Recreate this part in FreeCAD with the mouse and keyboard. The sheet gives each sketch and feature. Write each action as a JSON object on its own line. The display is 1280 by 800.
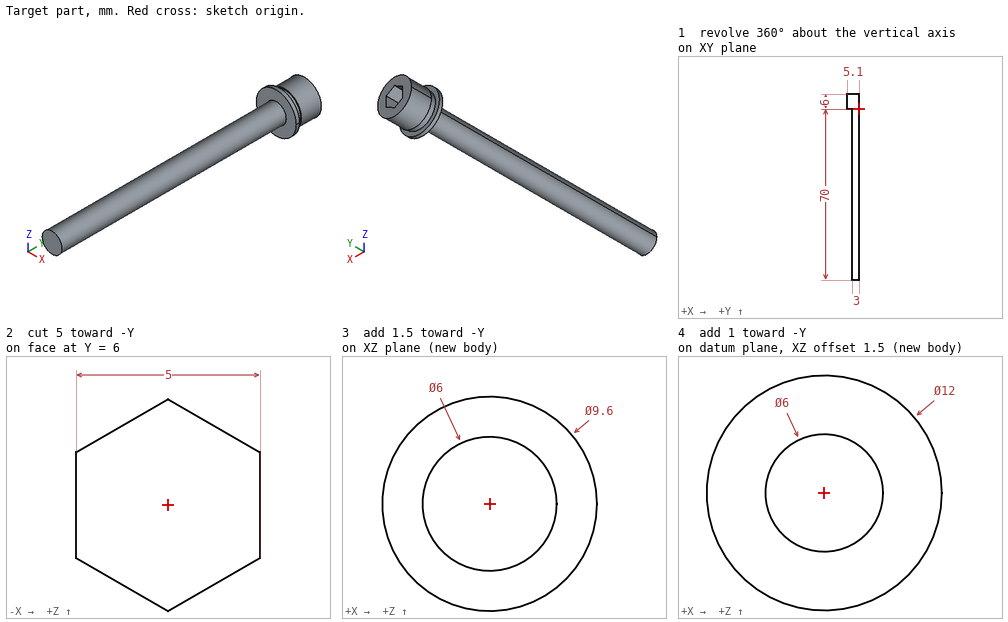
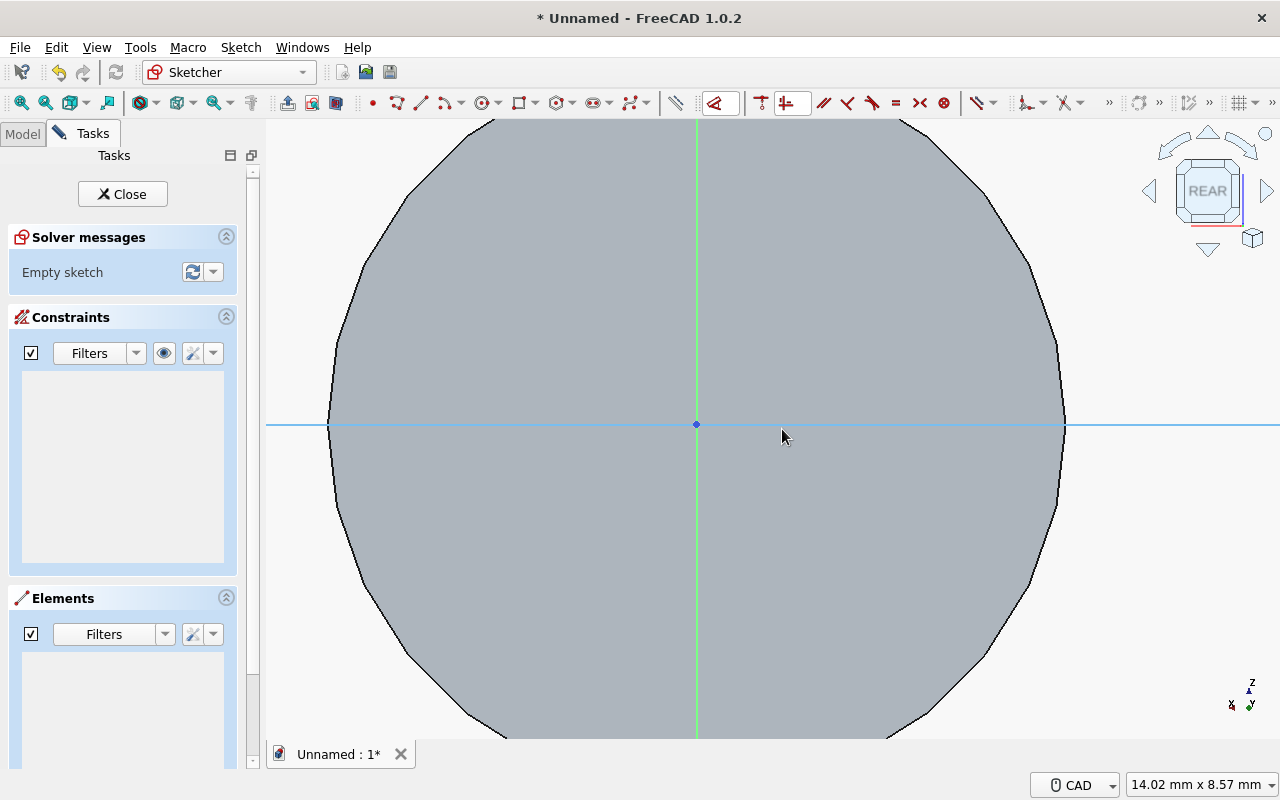
{"action": "key", "text": "g p 6"}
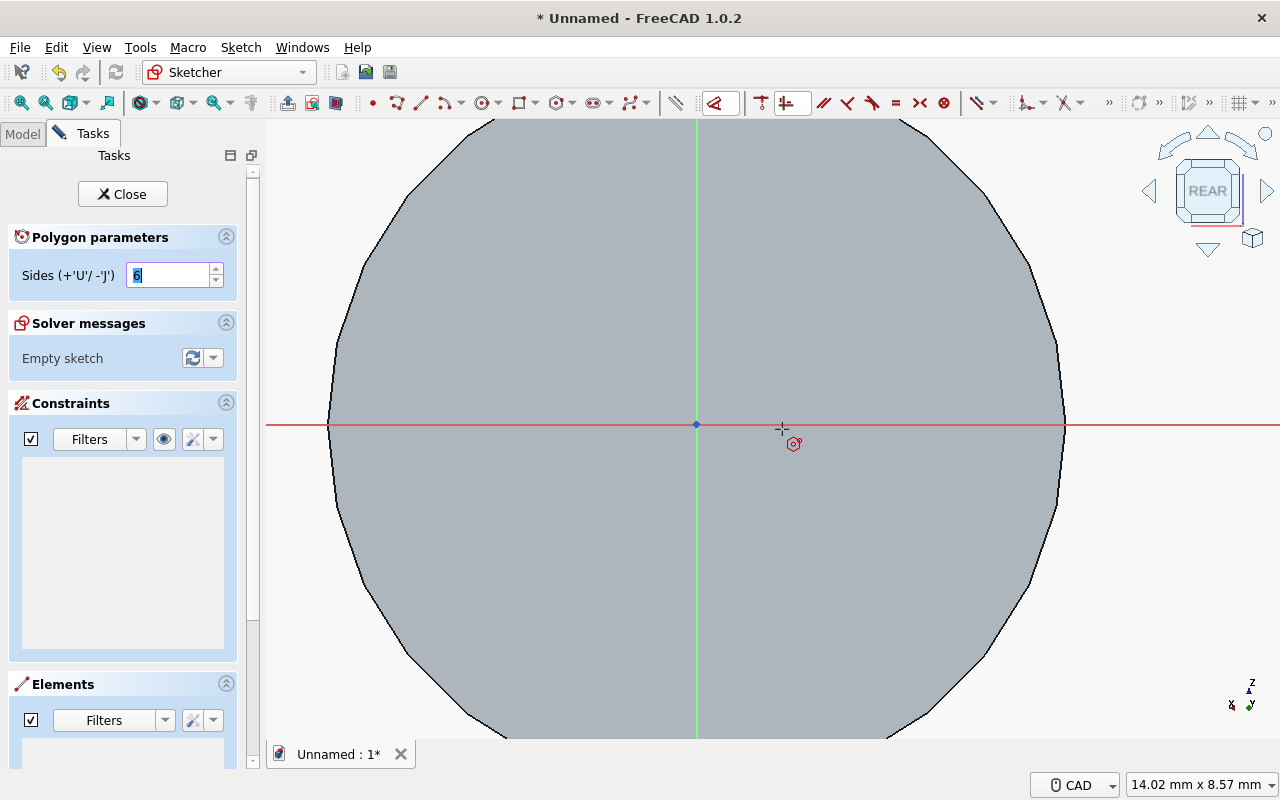
{"action": "left_click", "coordinate": [697, 425]}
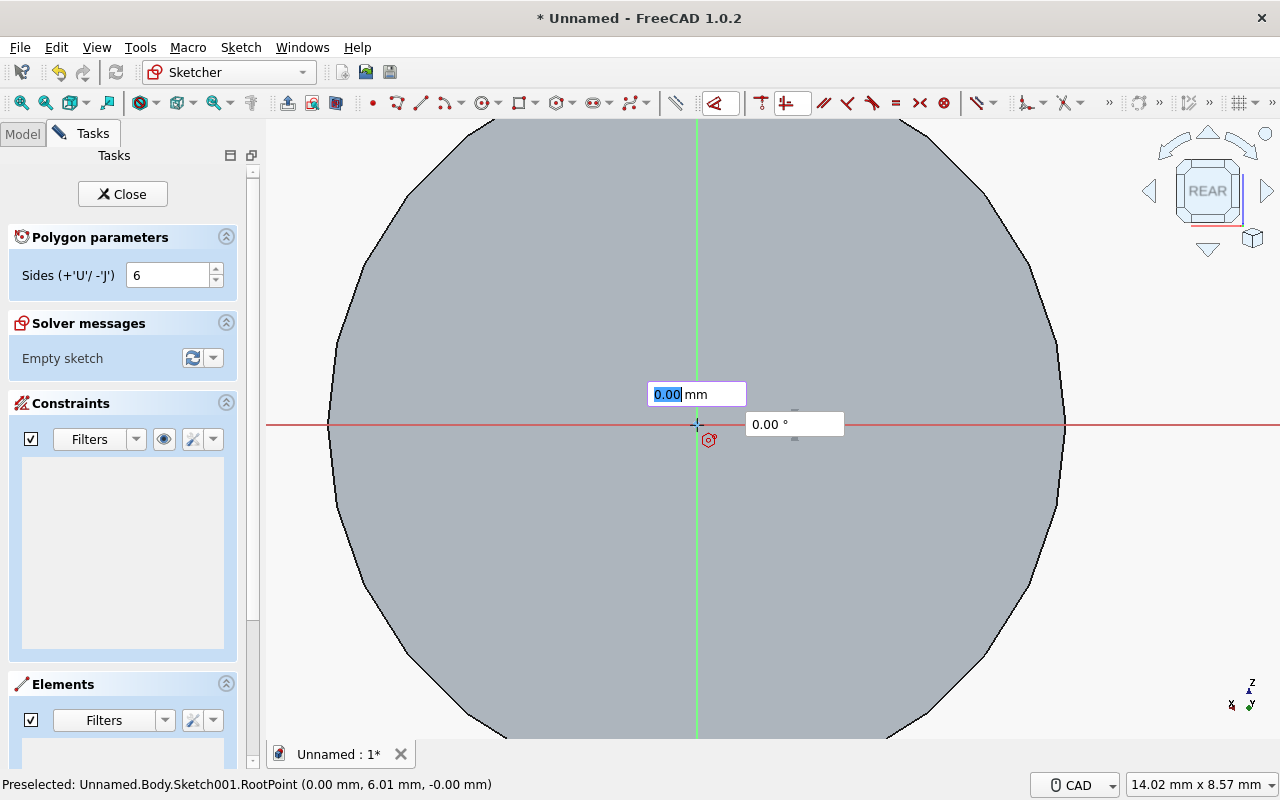
{"action": "left_click", "coordinate": [697, 634]}
{"action": "key", "text": "Escape"}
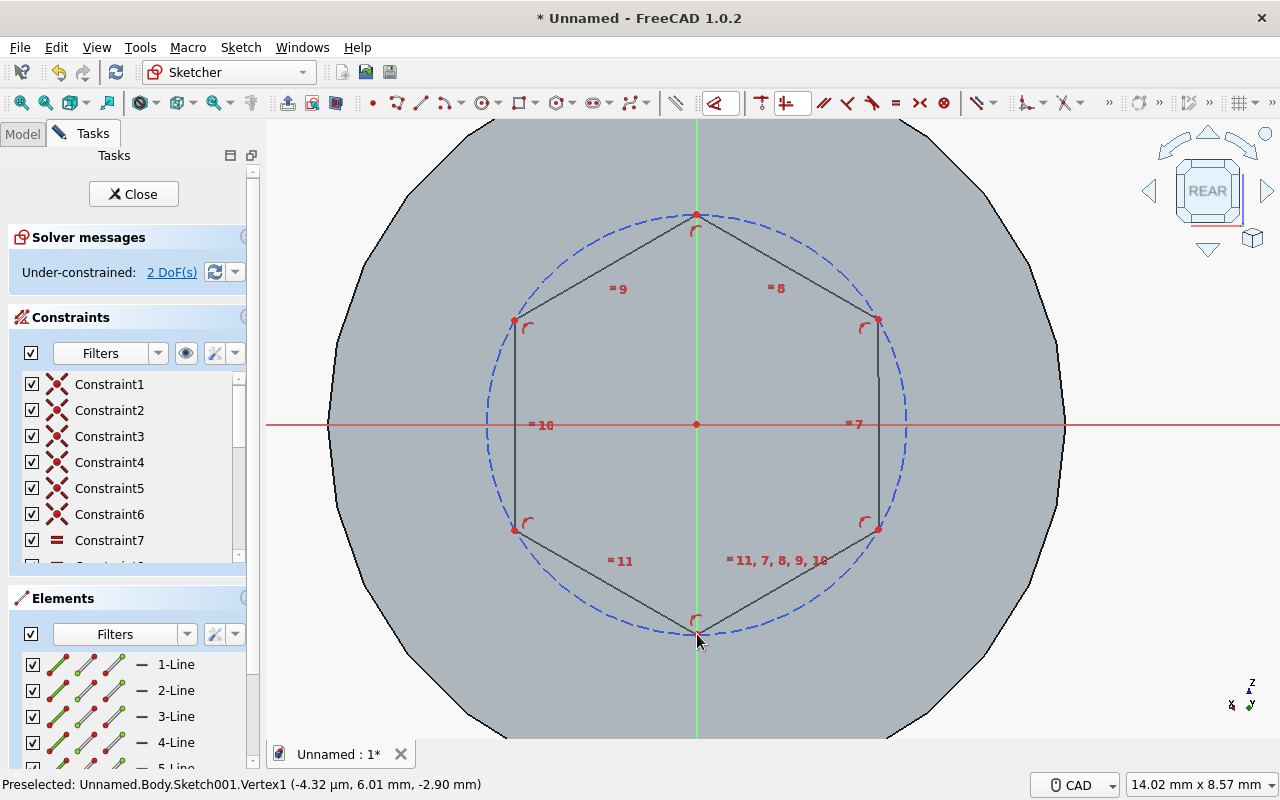
{"action": "left_click", "coordinate": [879, 467]}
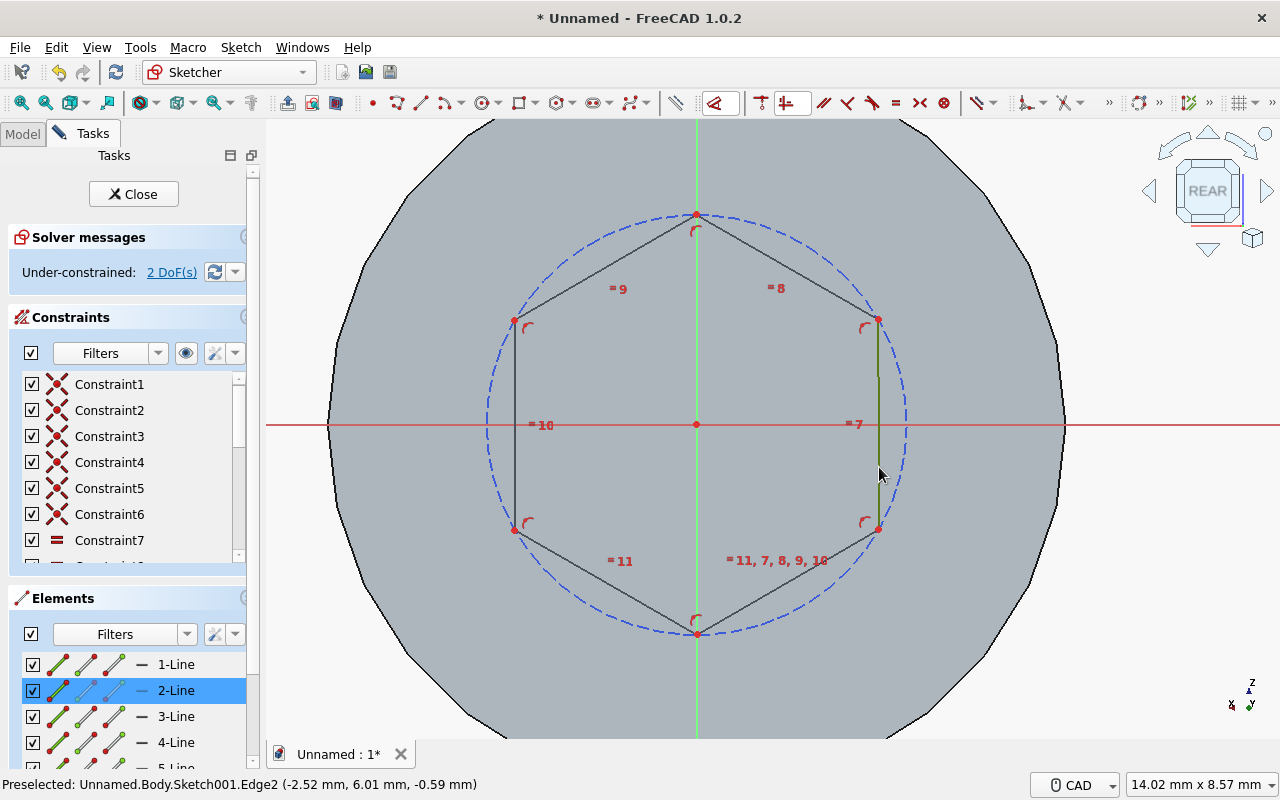
{"action": "key", "text": "v"}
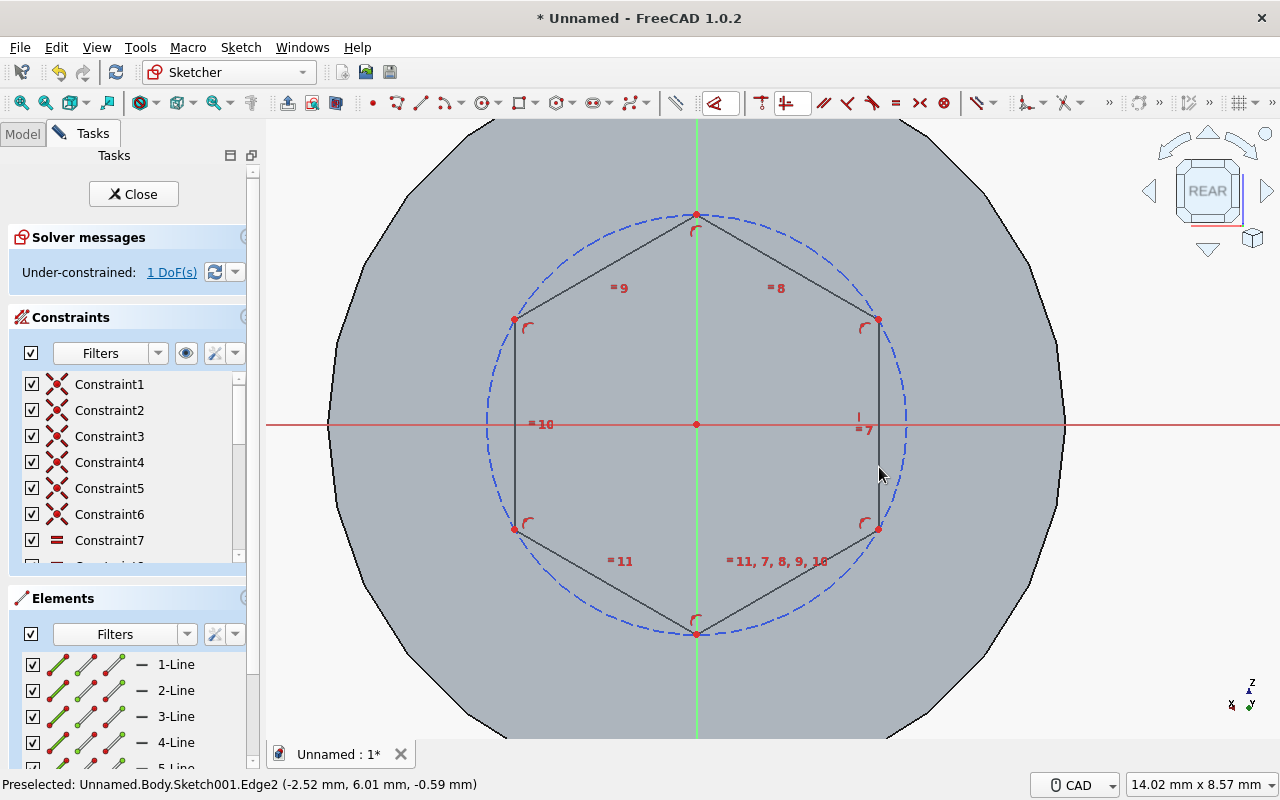
{"action": "left_click", "coordinate": [515, 320]}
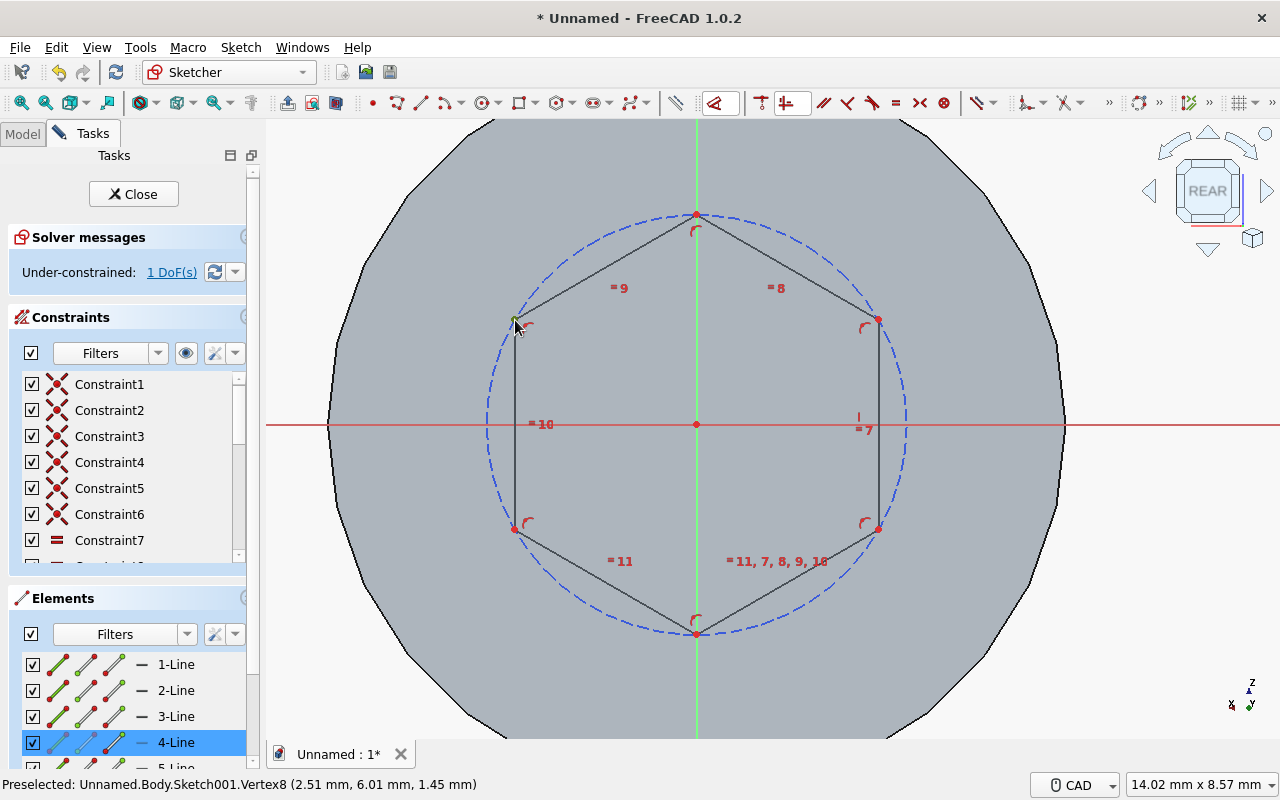
{"action": "left_click", "coordinate": [879, 530]}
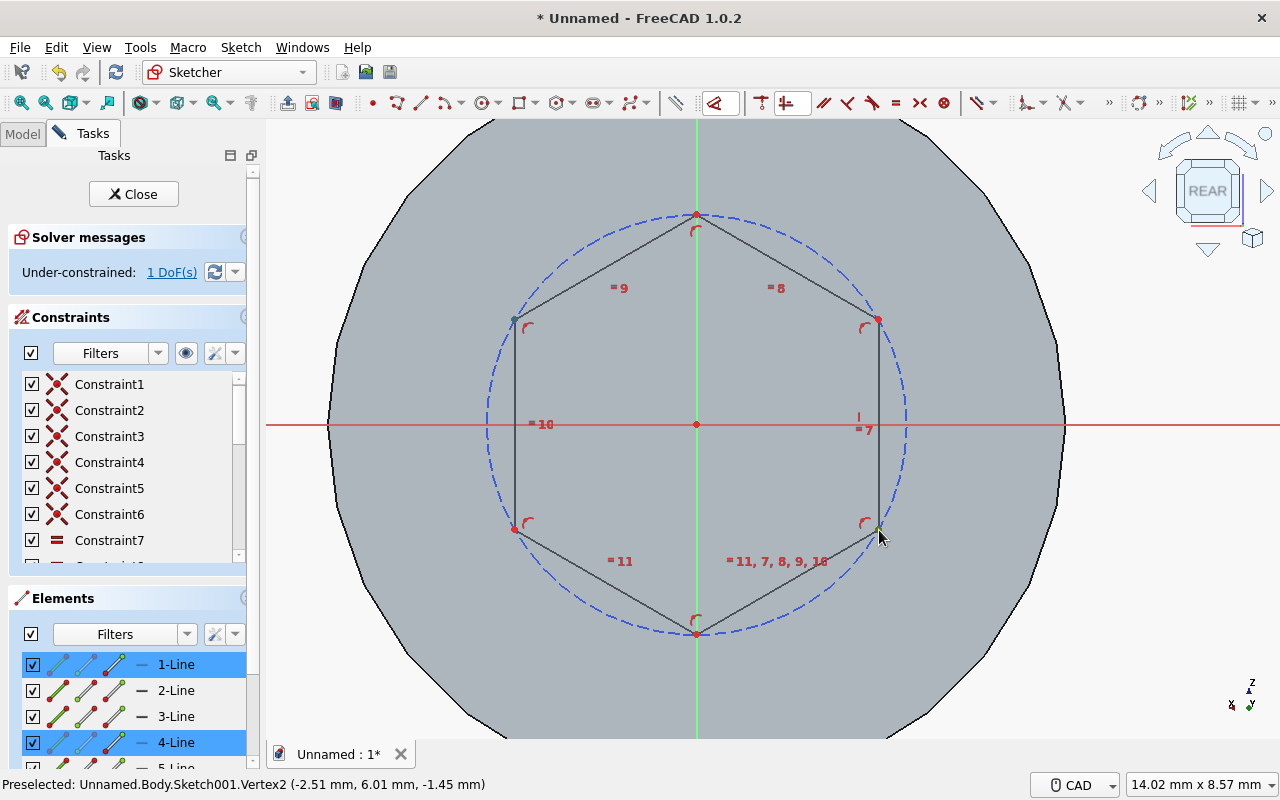
{"action": "key", "text": "l"}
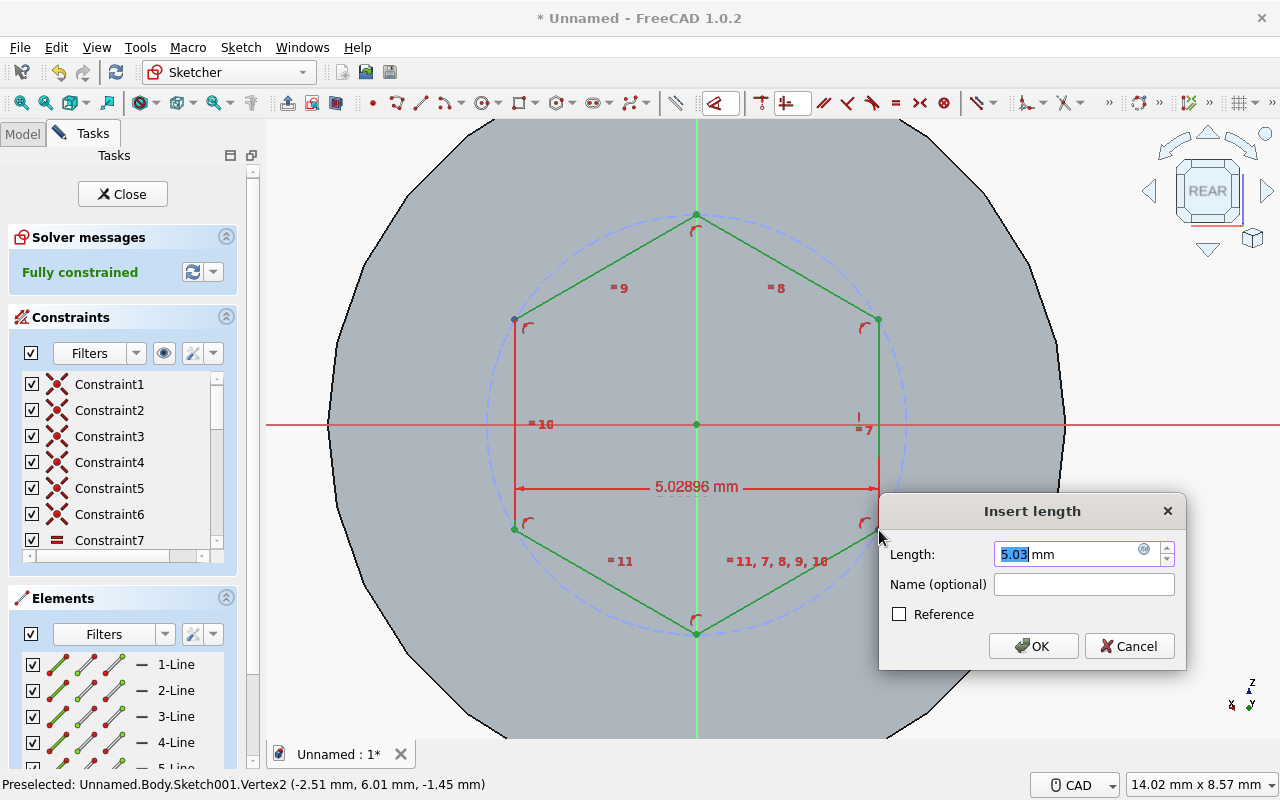
{"action": "type", "text": "5"}
{"action": "key", "text": "Return"}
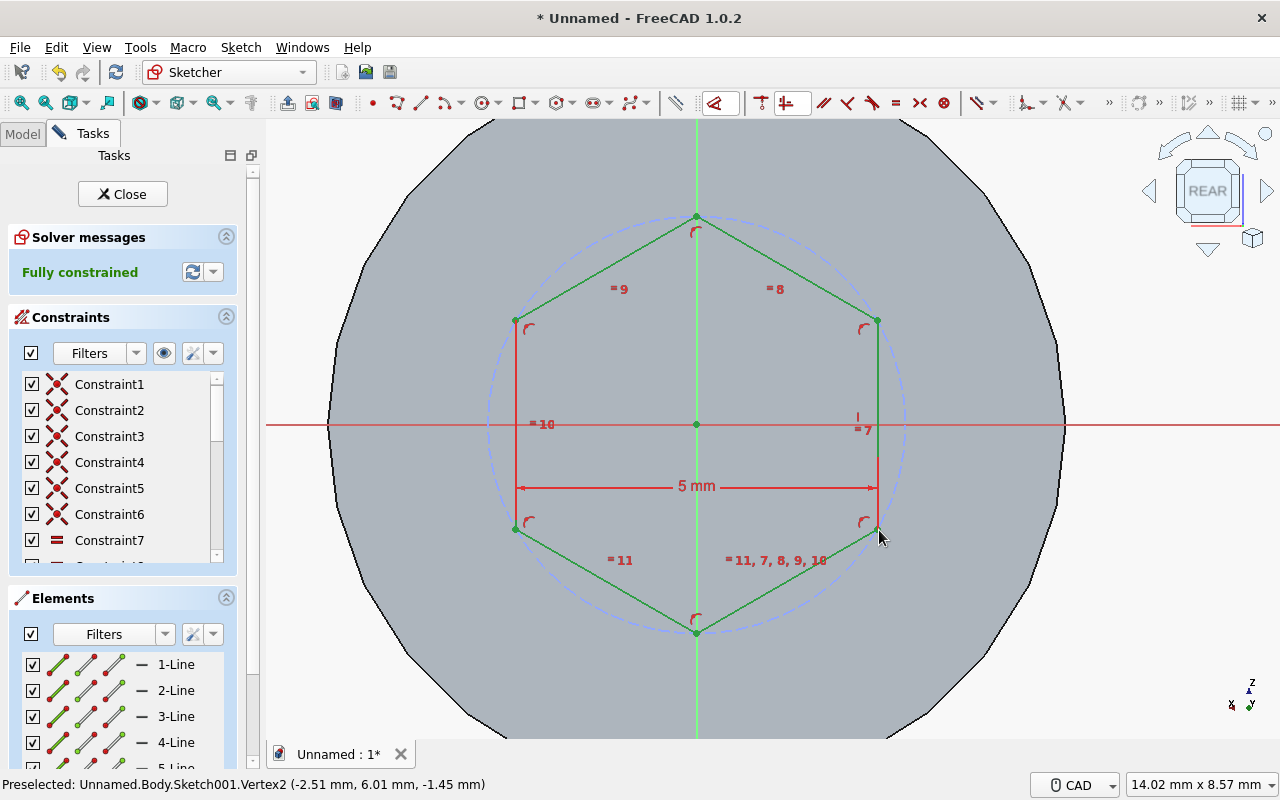
{"action": "left_click", "coordinate": [123, 194]}